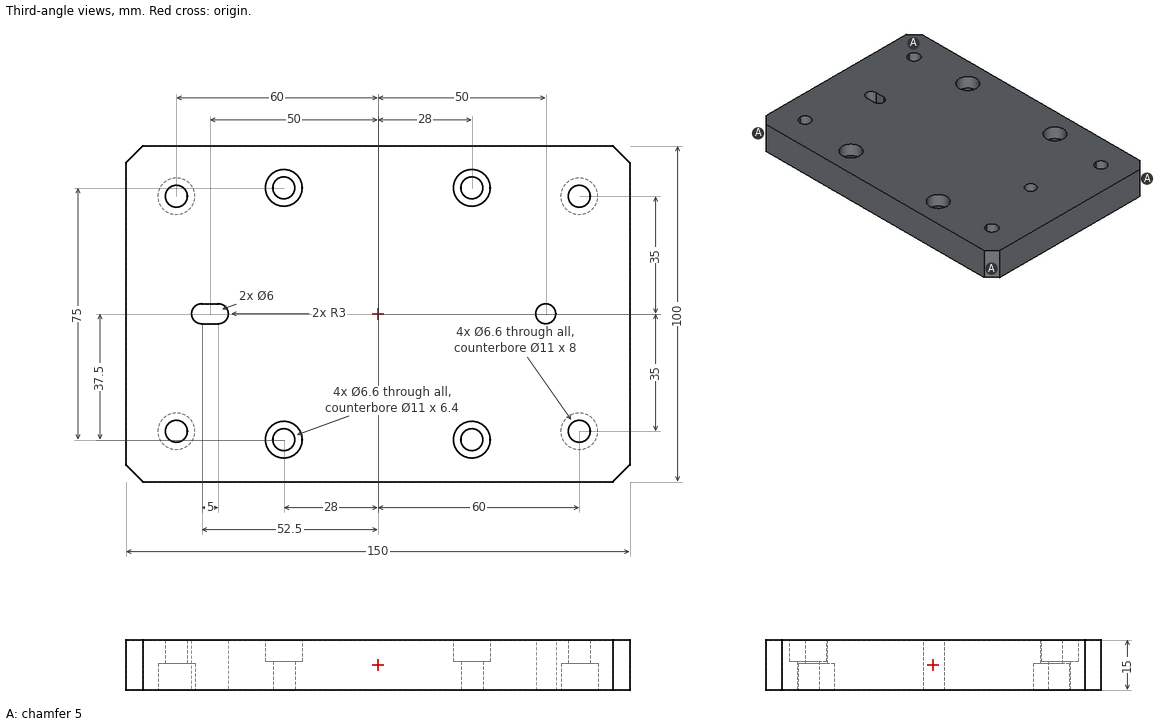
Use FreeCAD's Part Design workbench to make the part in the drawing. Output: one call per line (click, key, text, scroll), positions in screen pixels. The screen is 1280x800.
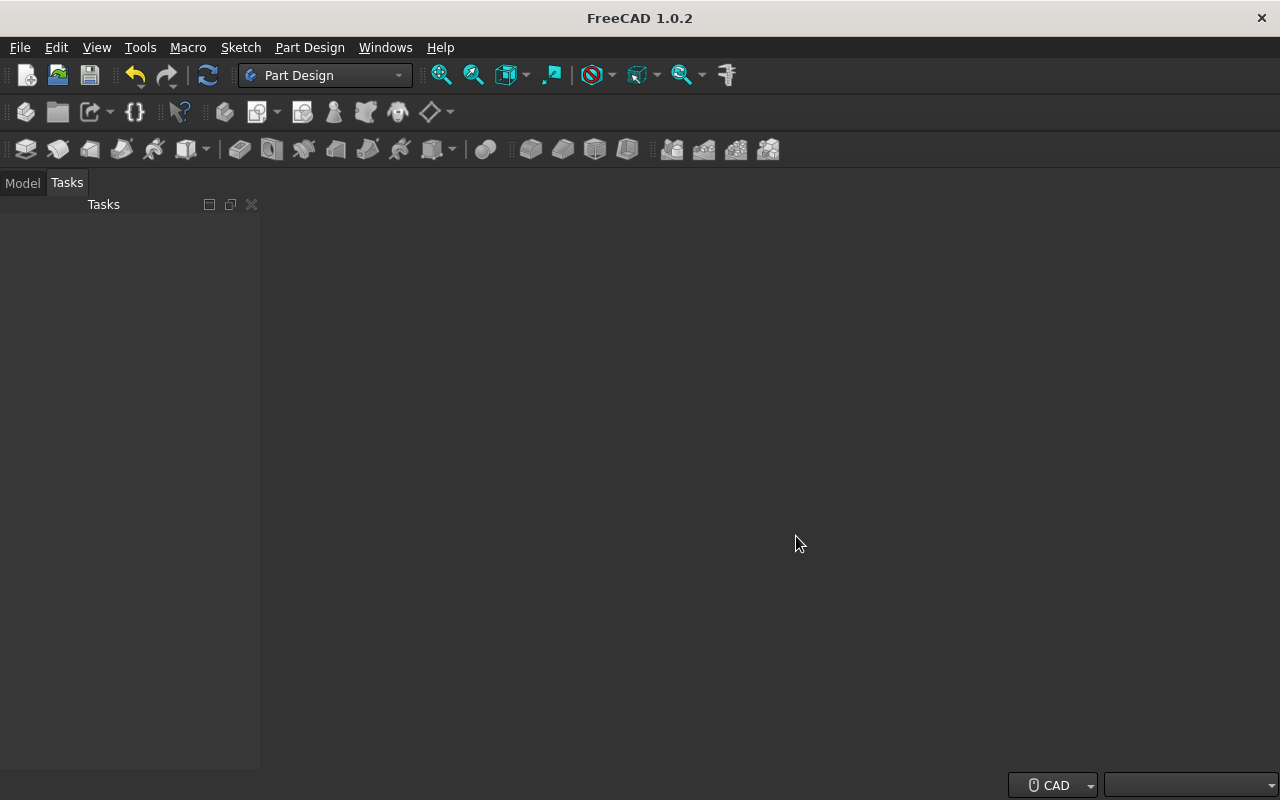
click(26, 76)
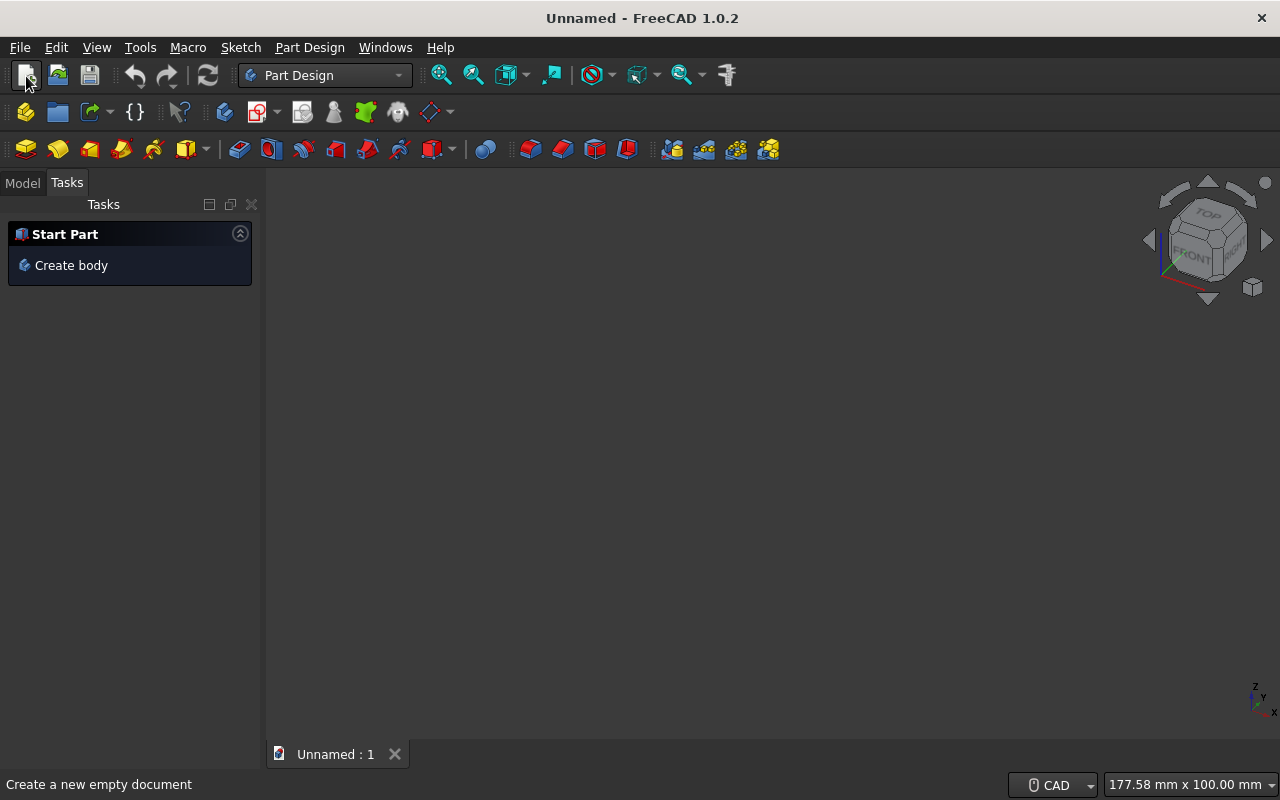
click(258, 112)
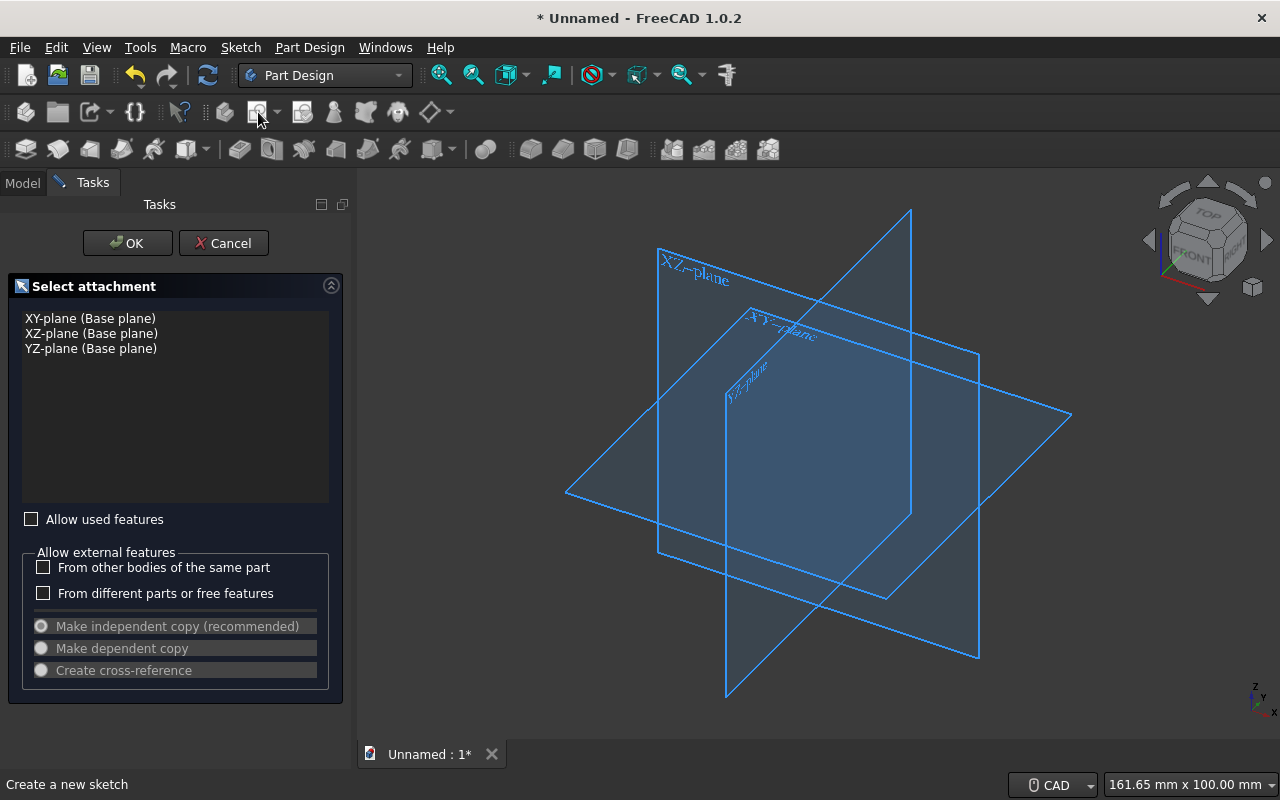
click(82, 318)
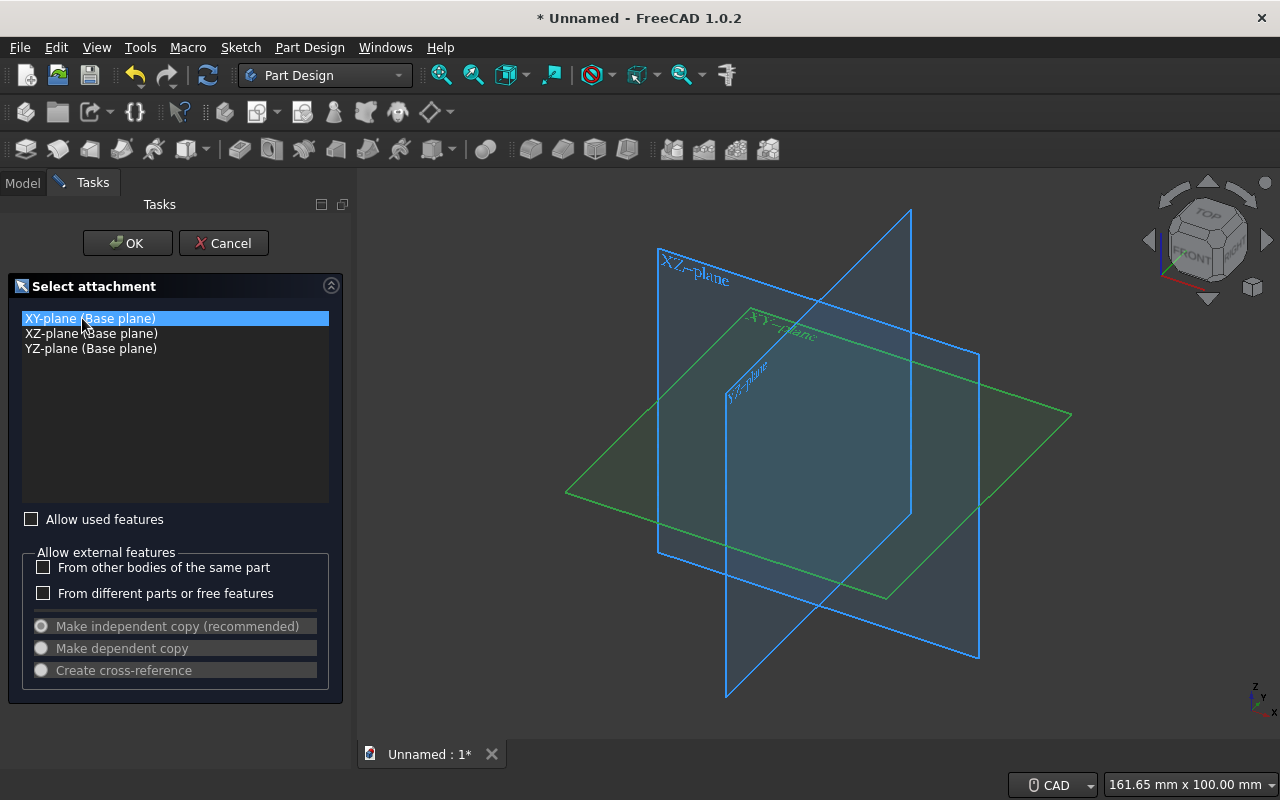
click(128, 243)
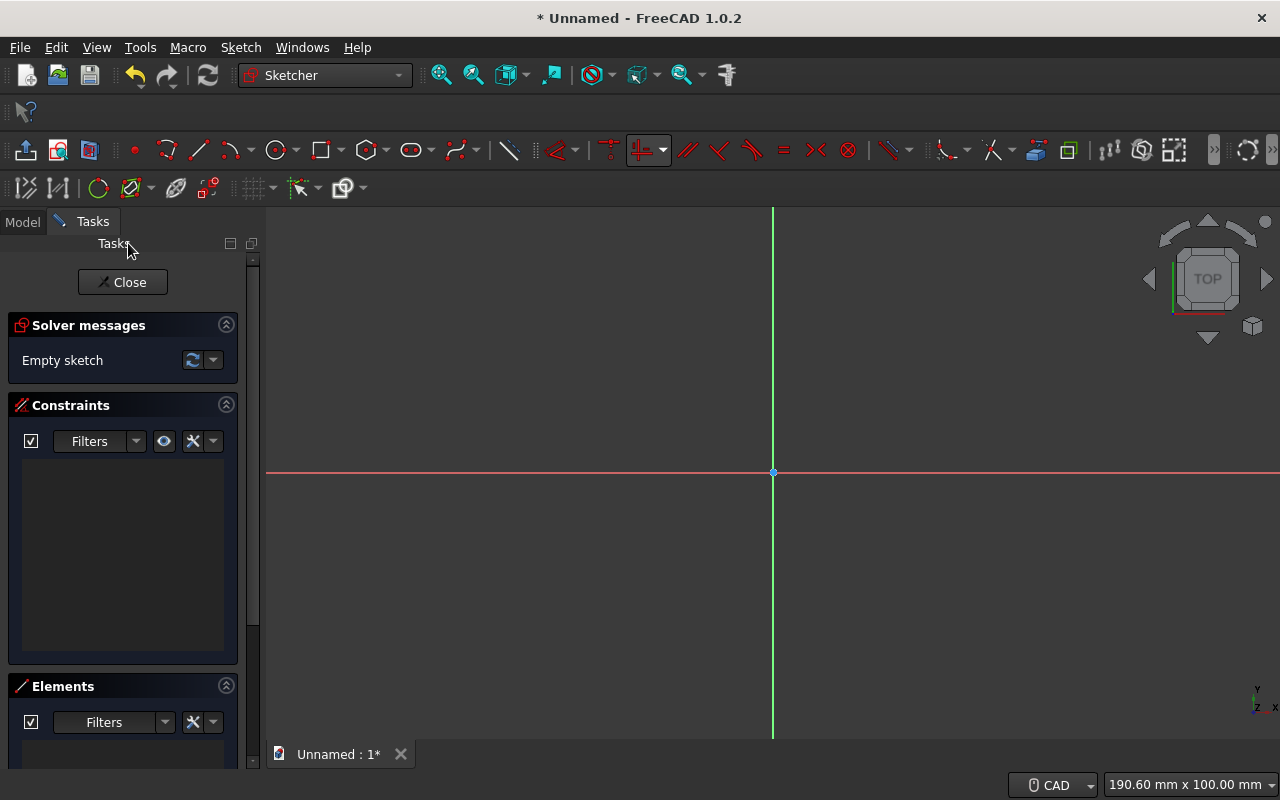
scroll(565, 473, down, 2)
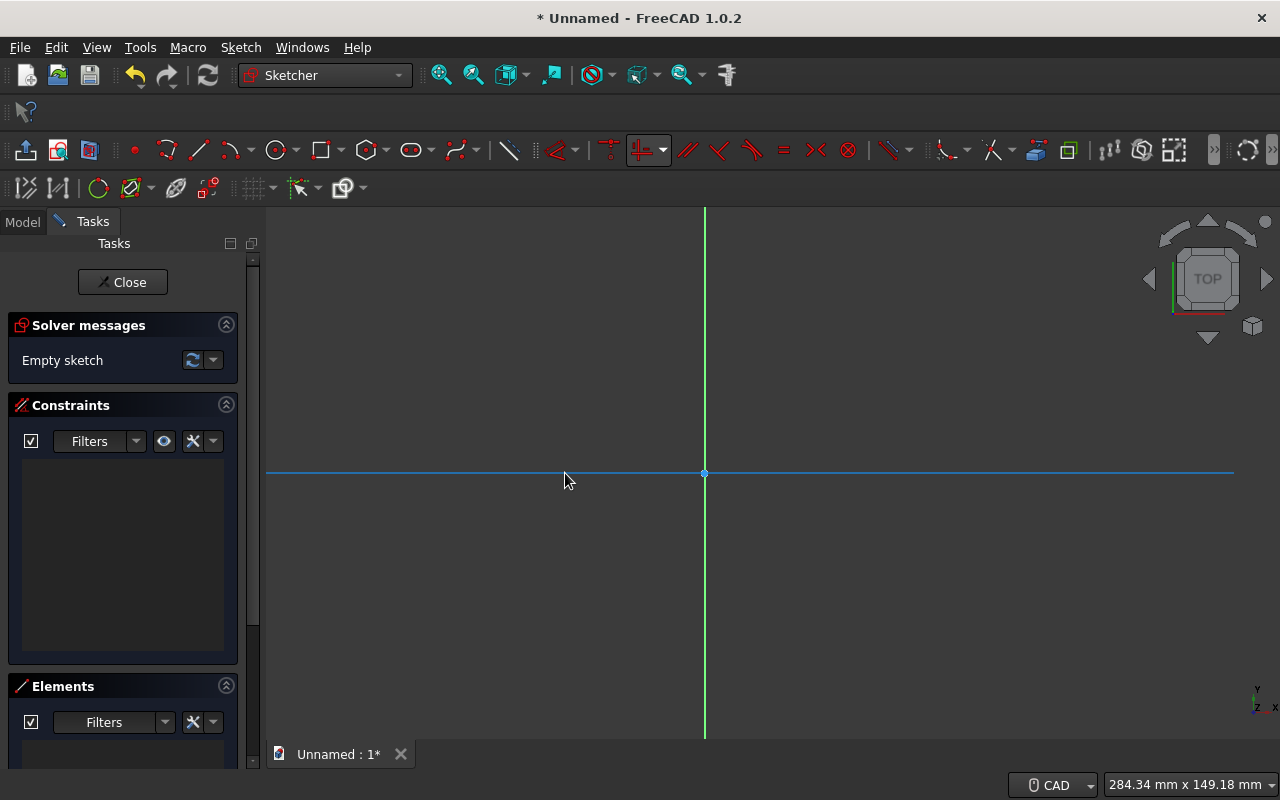
key(g)
key(v)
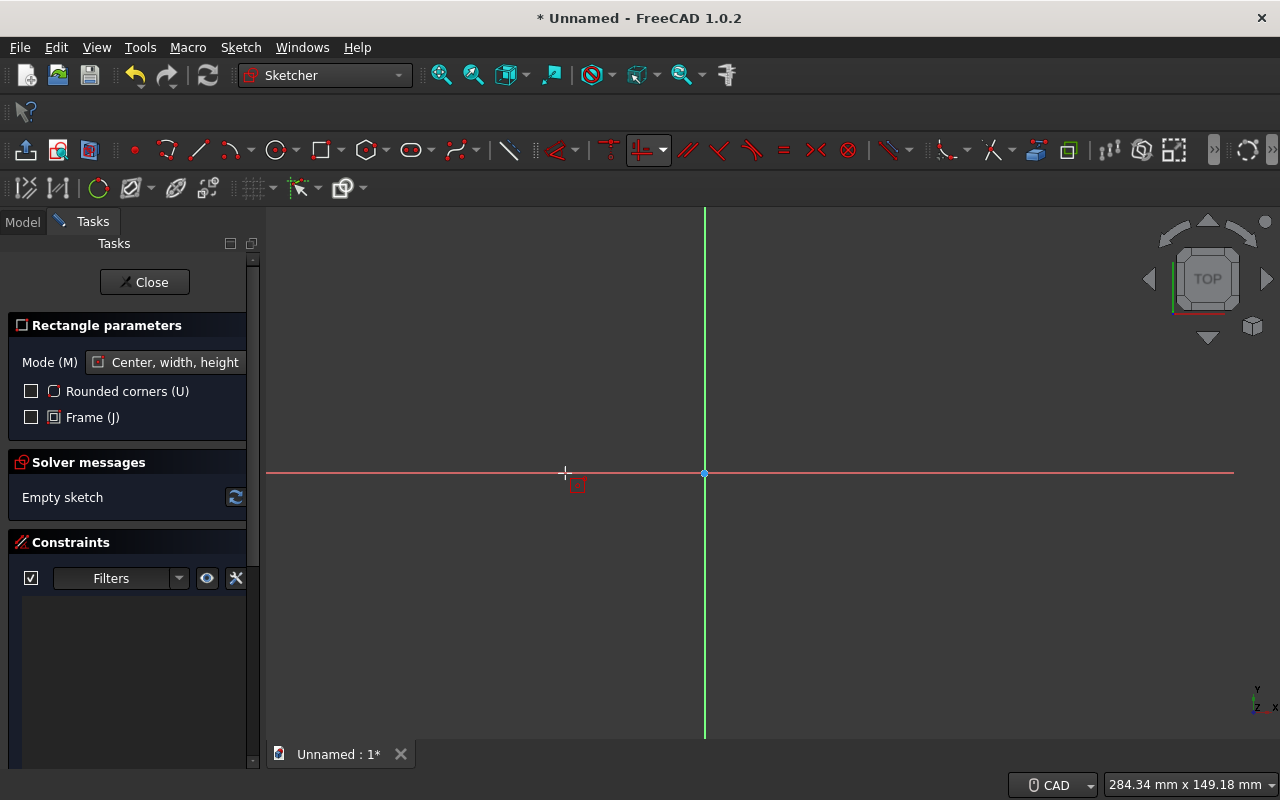
click(705, 473)
move(972, 295)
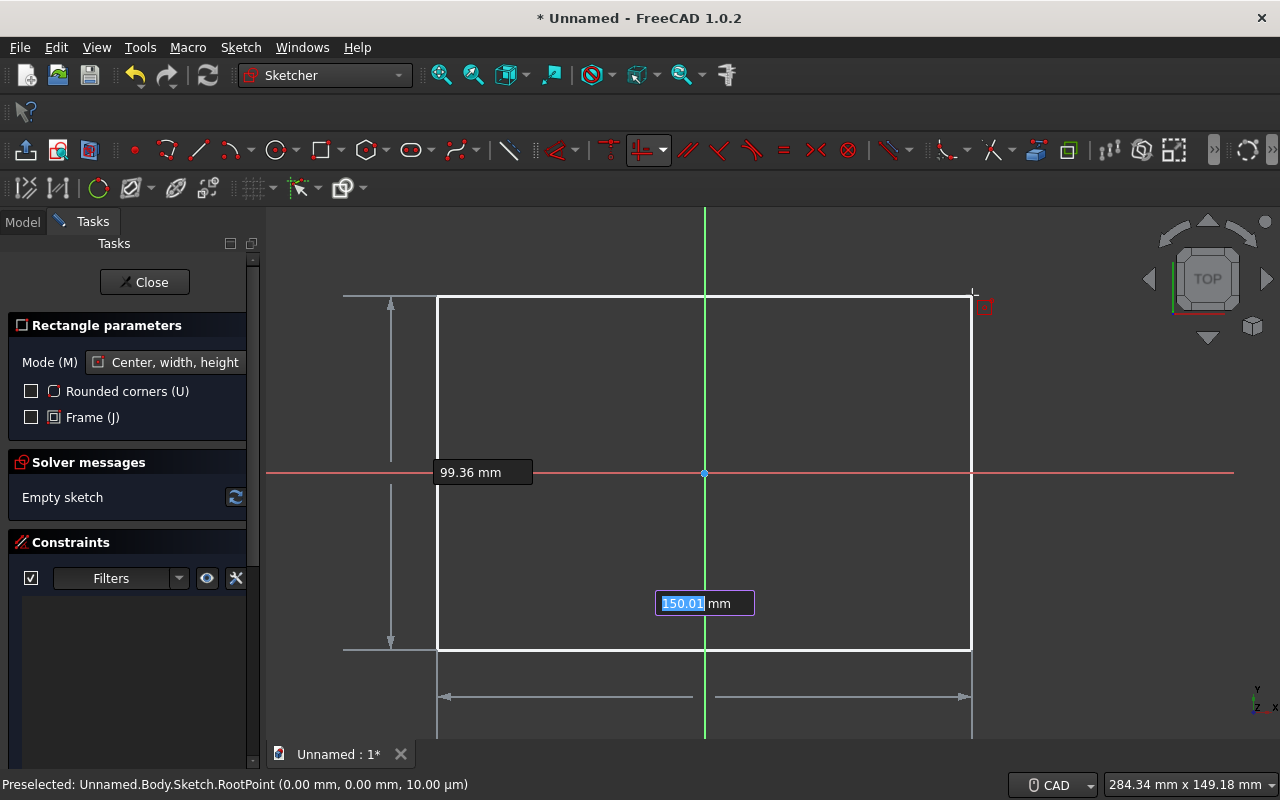
text(150)
key(Tab)
text(100)
key(Return)
key(Escape)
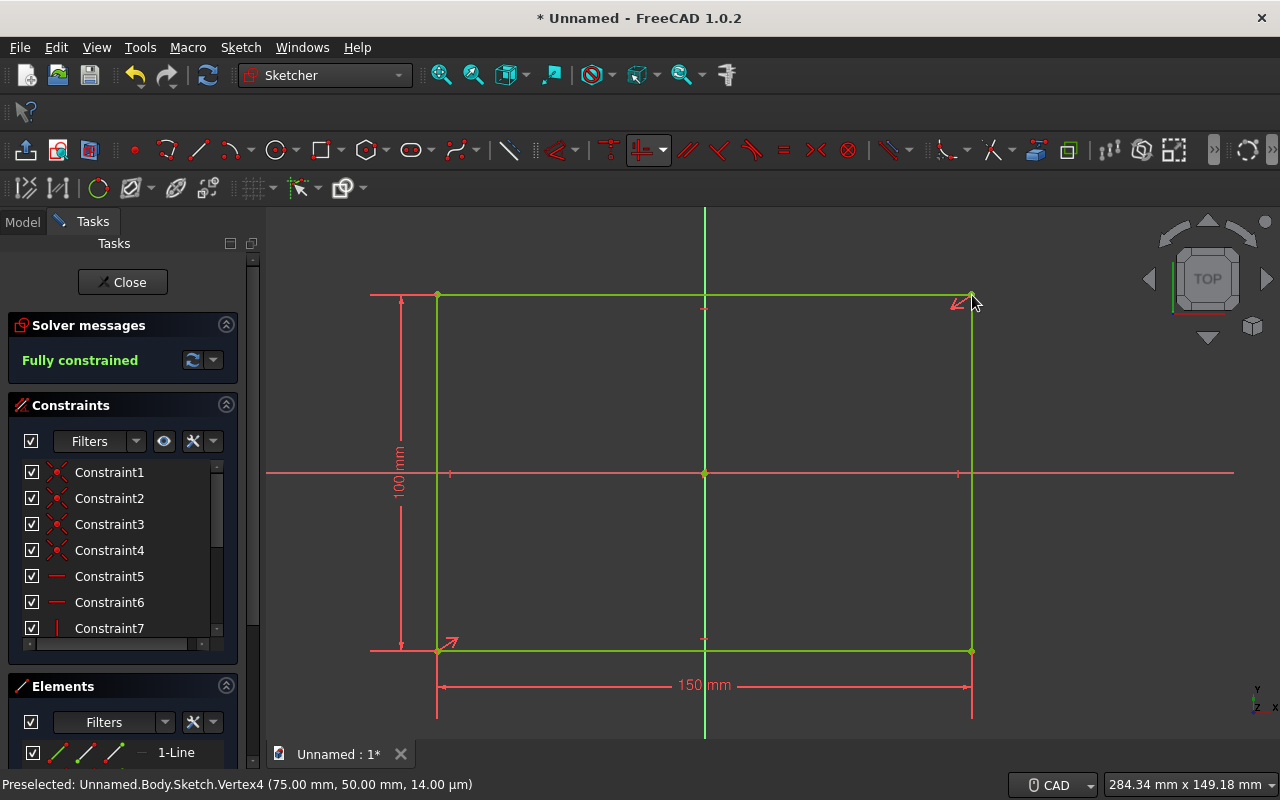
click(123, 282)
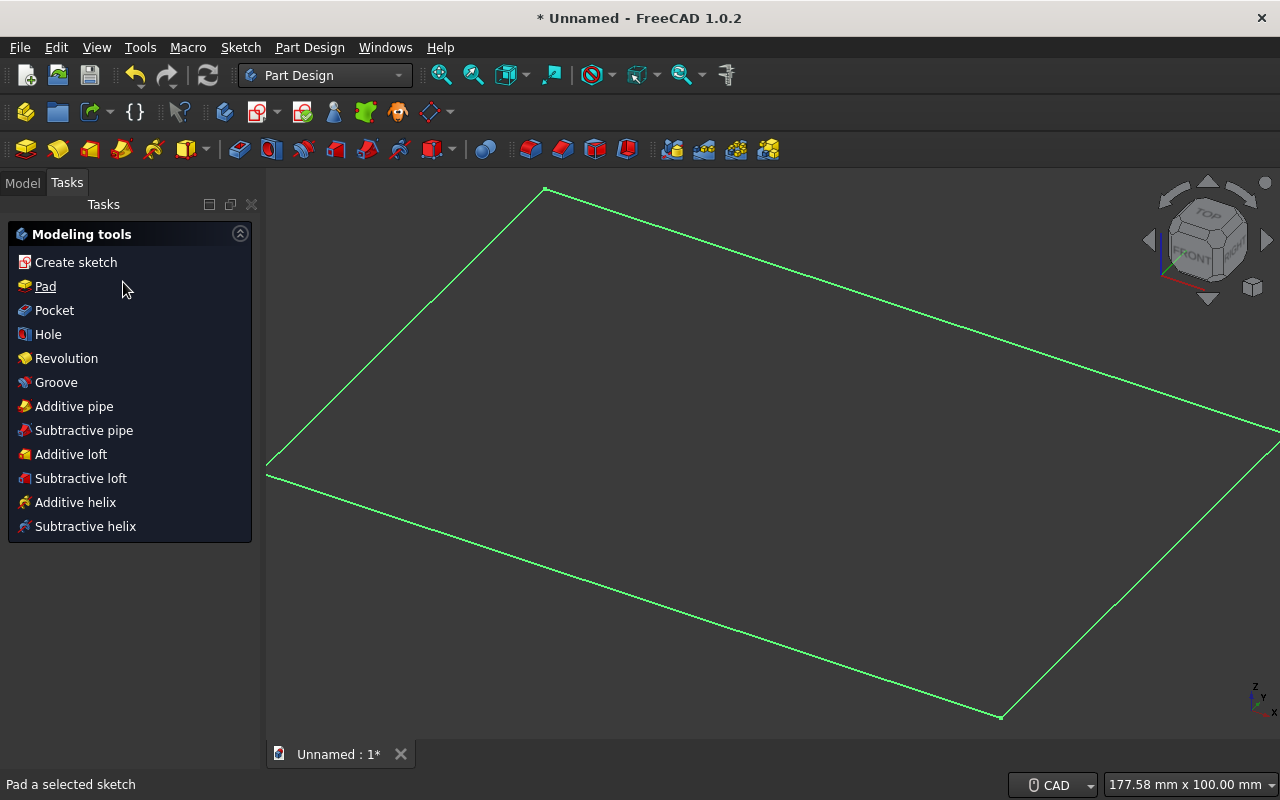
click(26, 150)